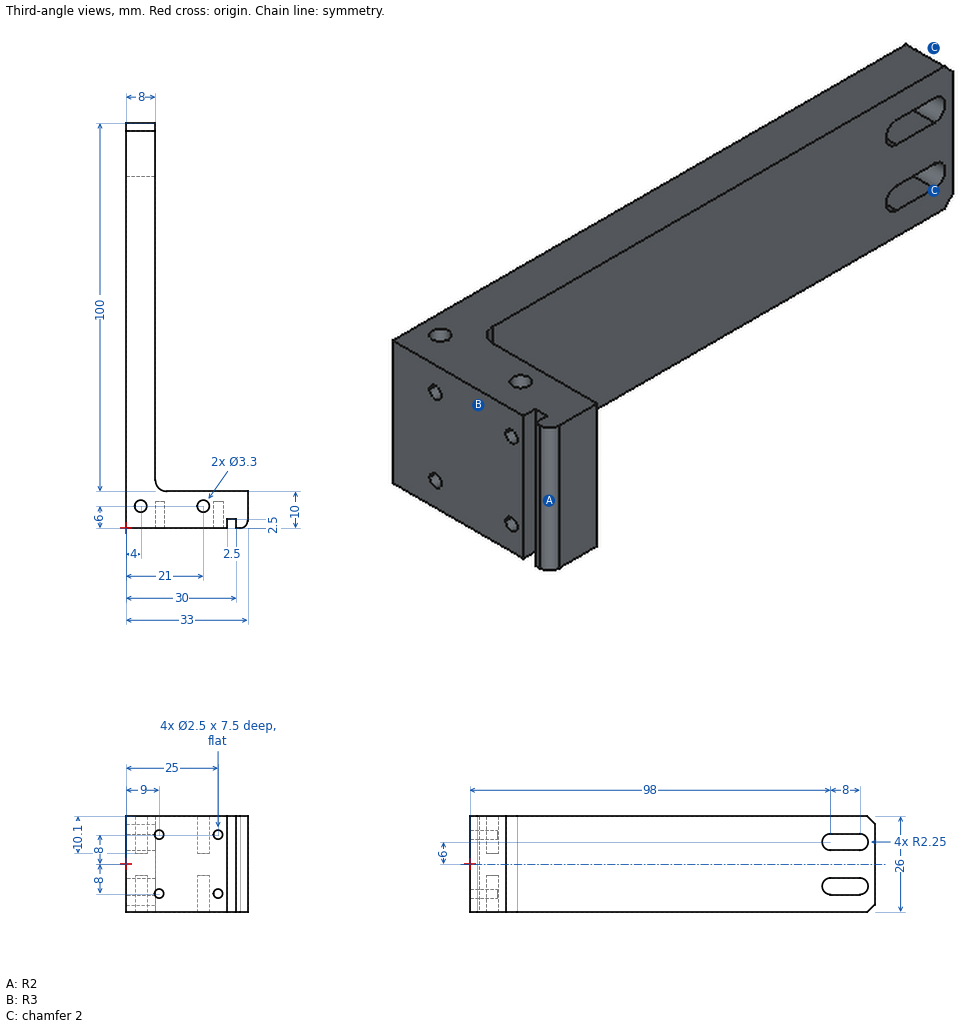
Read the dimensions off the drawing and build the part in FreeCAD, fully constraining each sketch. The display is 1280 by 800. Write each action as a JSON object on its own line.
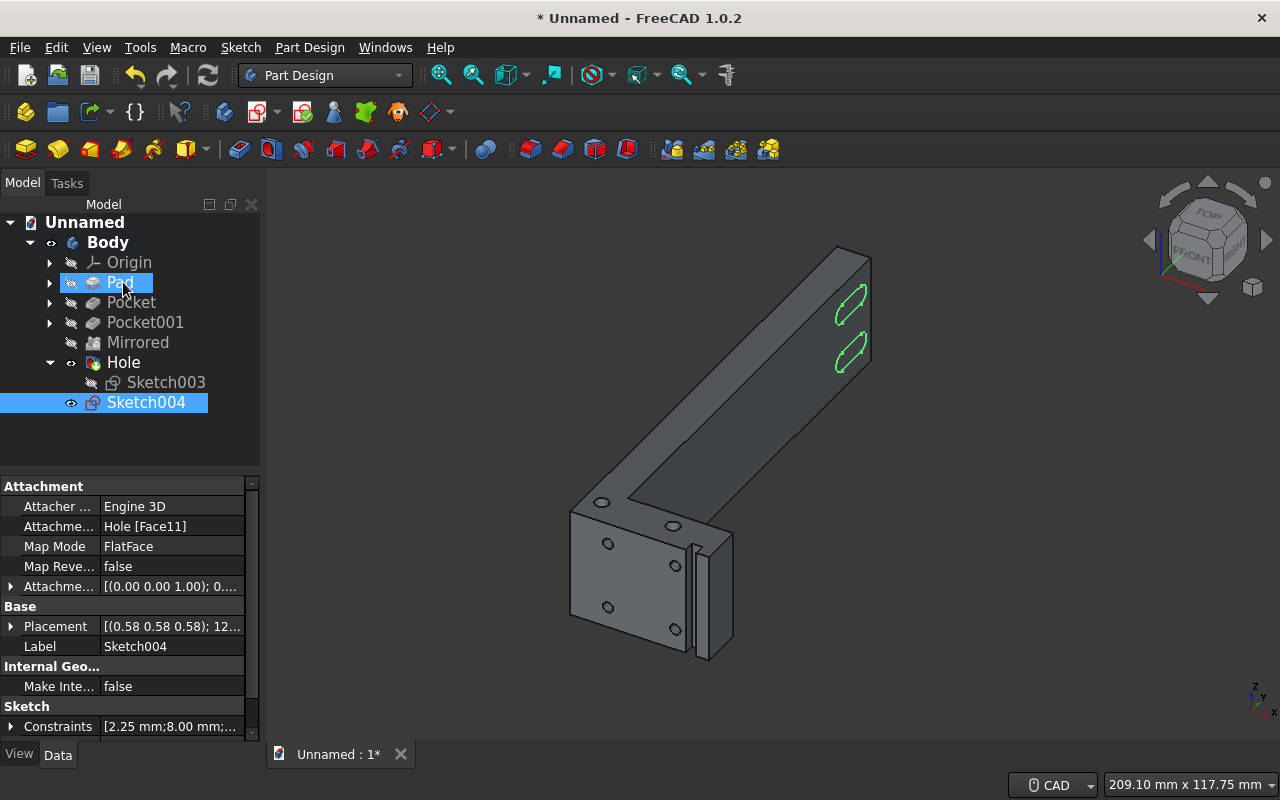
{"action": "left_click", "coordinate": [240, 150]}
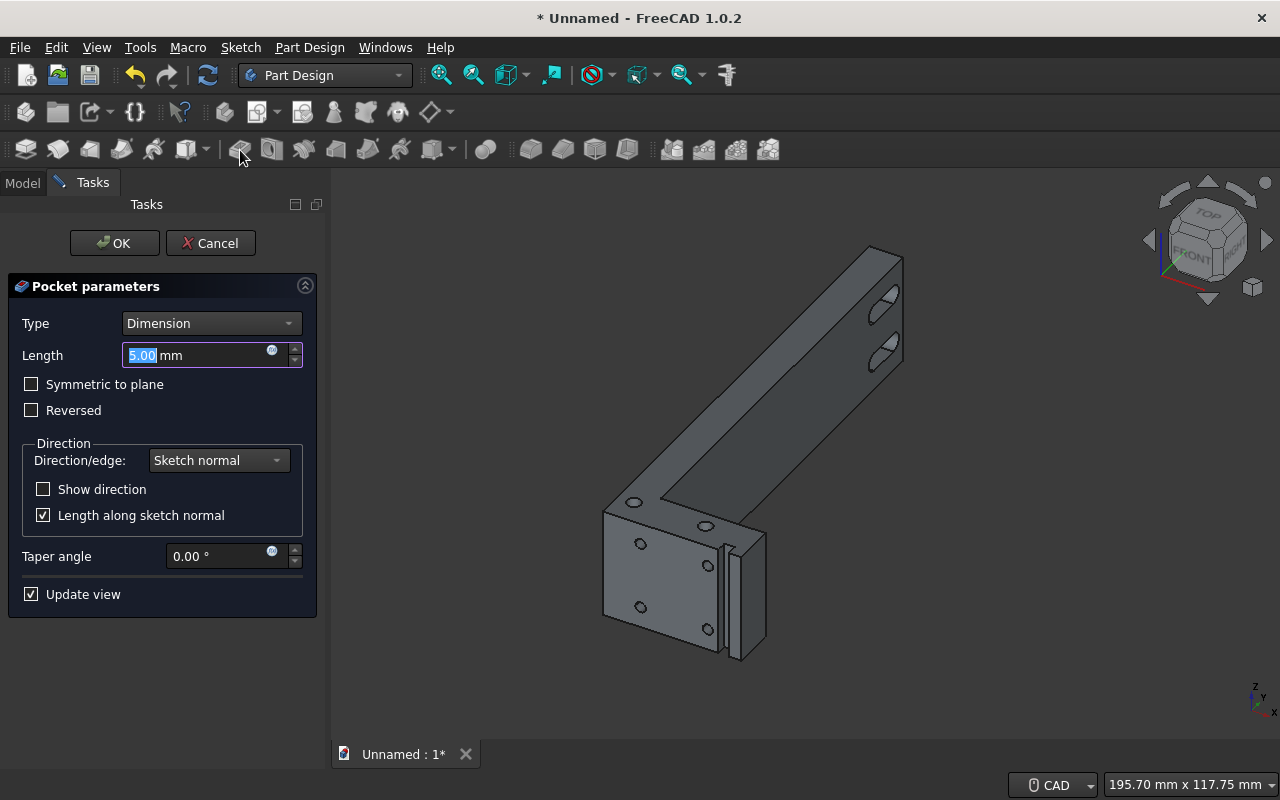
{"action": "left_click", "coordinate": [212, 324]}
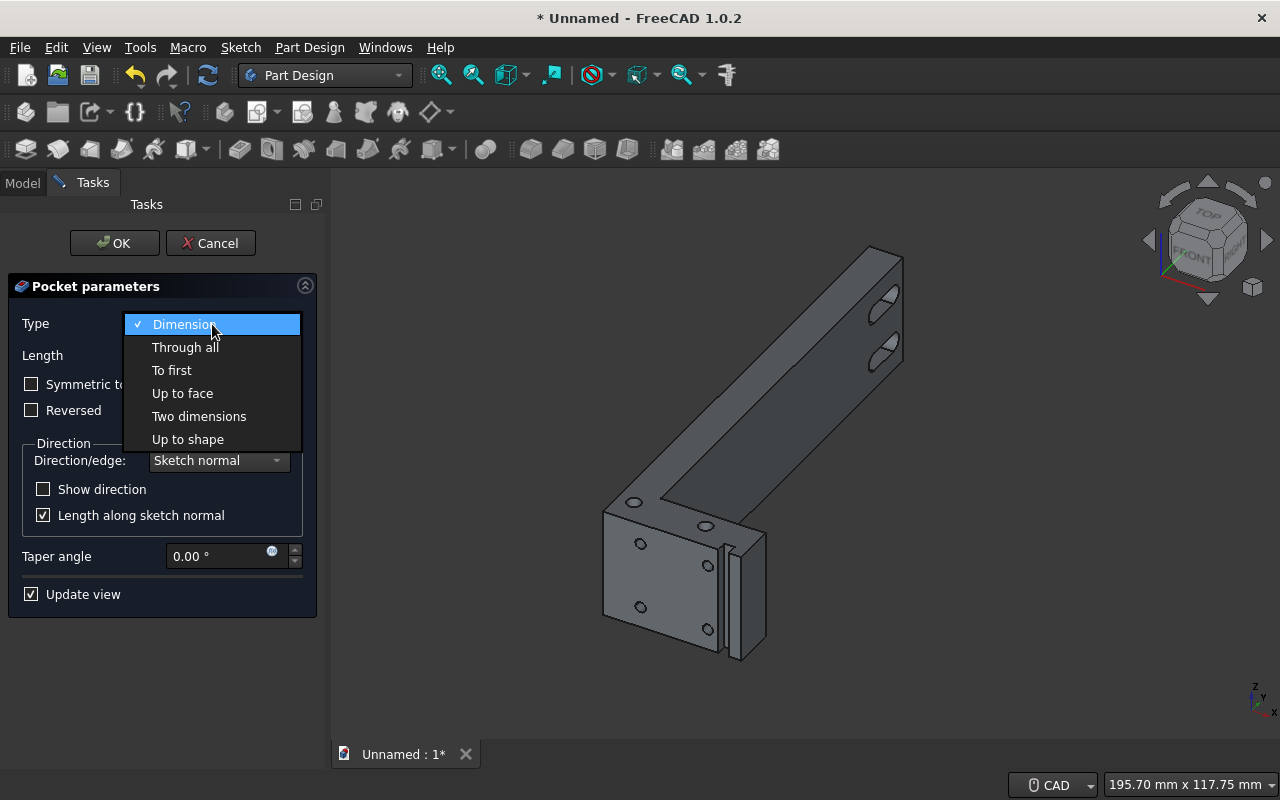
{"action": "left_click", "coordinate": [212, 348]}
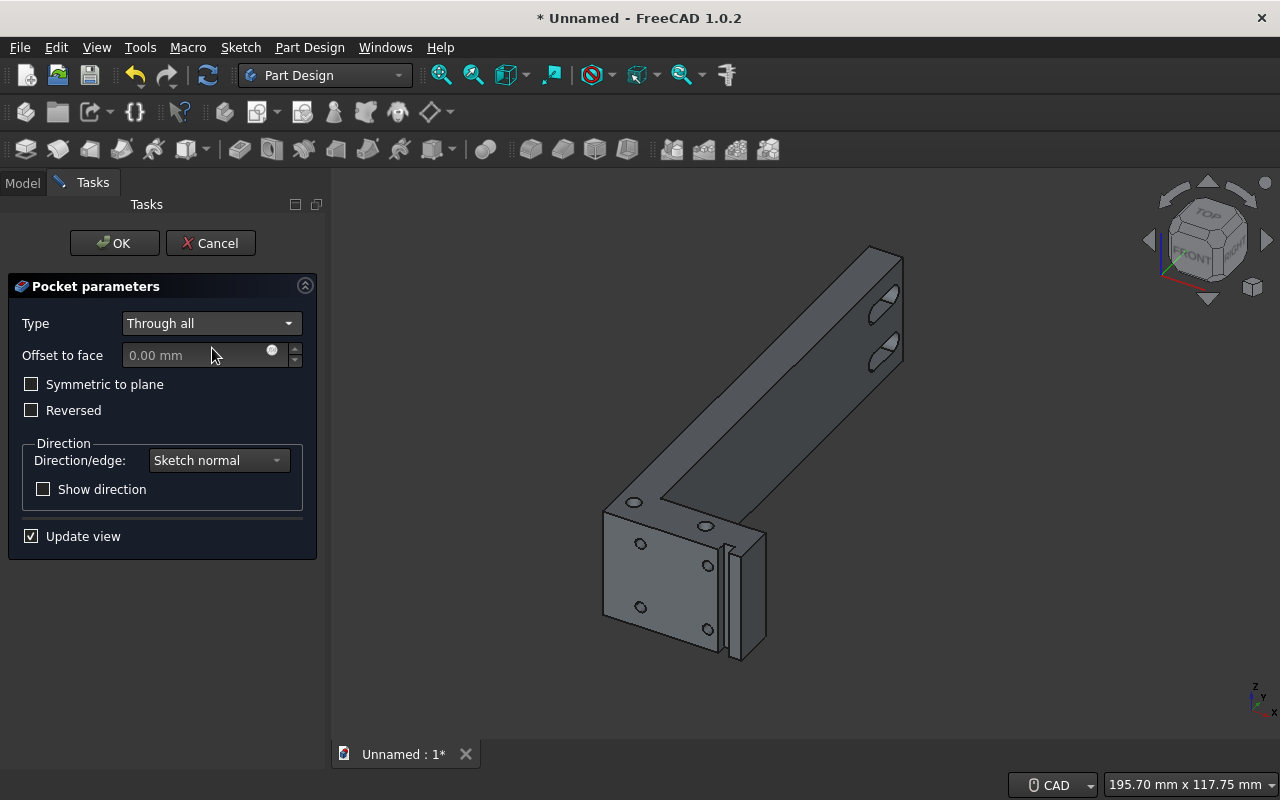
{"action": "left_click", "coordinate": [115, 243]}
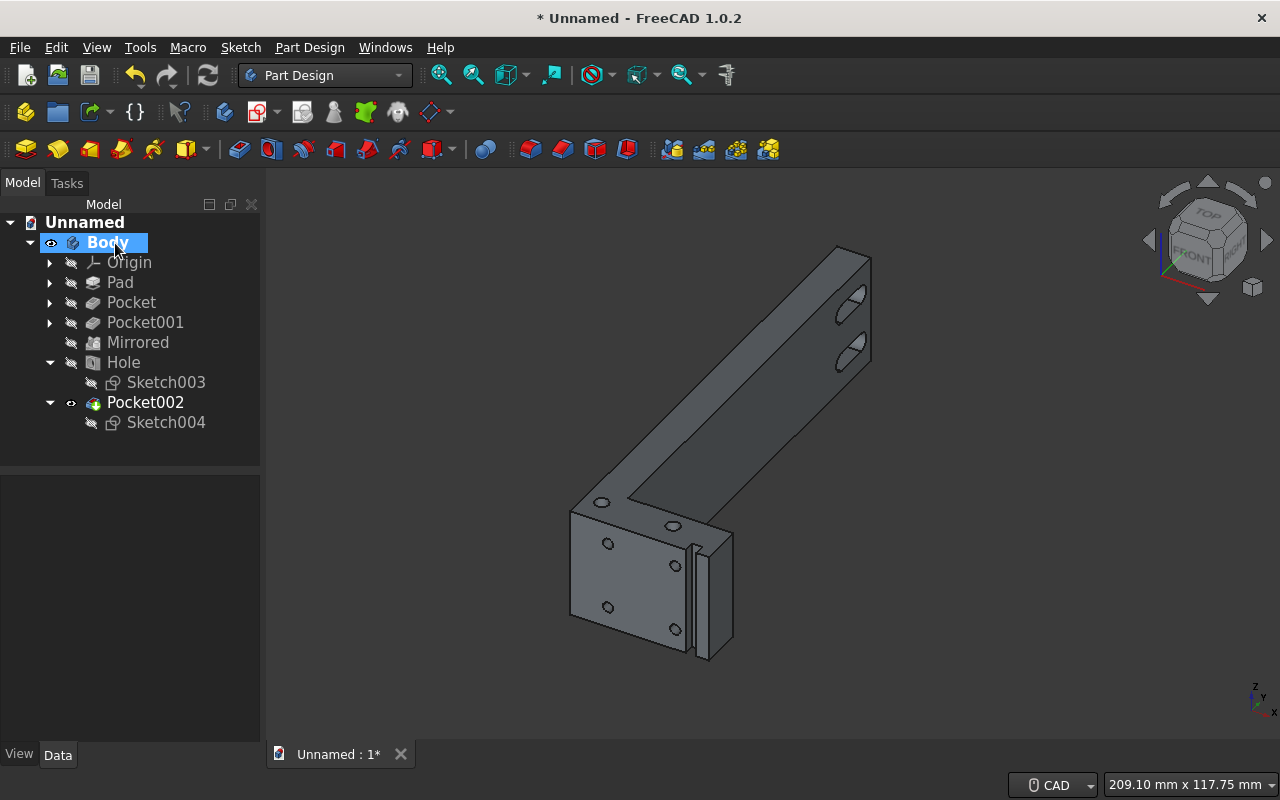
{"action": "left_click", "coordinate": [709, 608]}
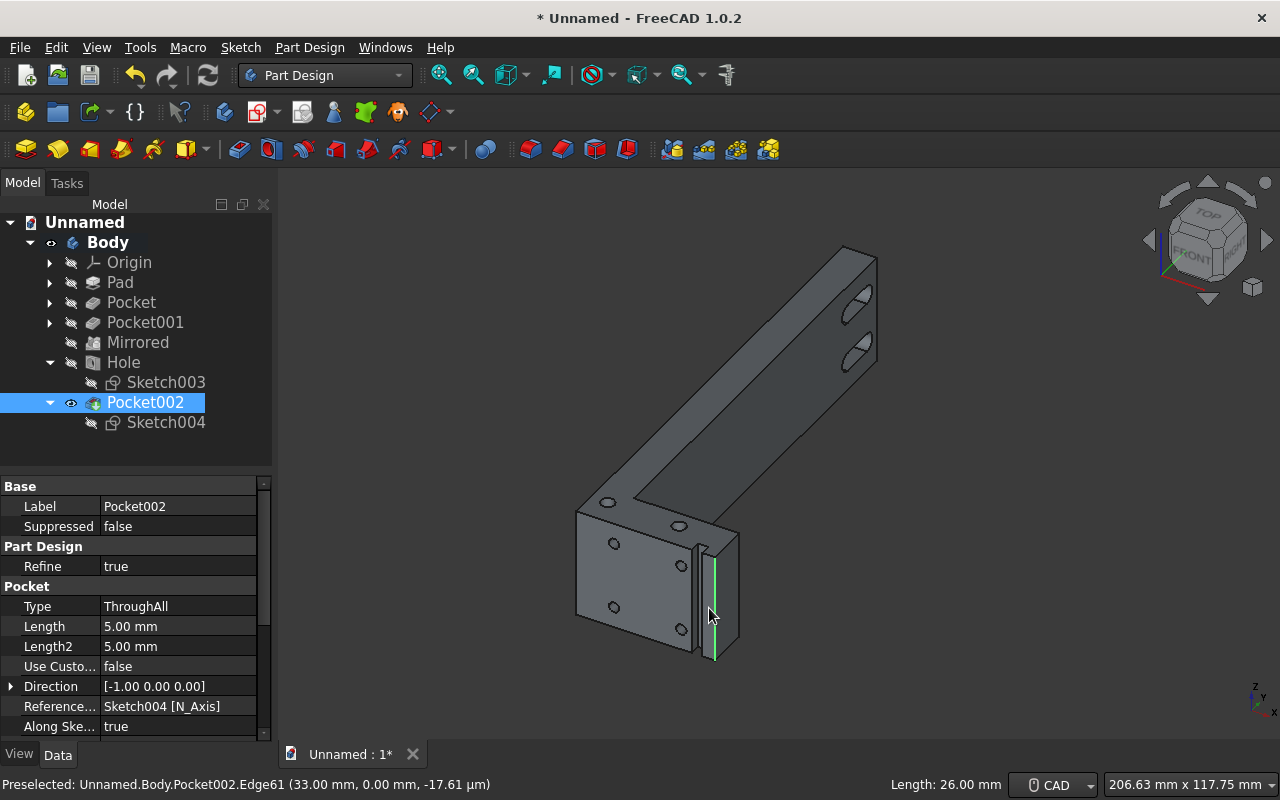
{"action": "left_click", "coordinate": [532, 150]}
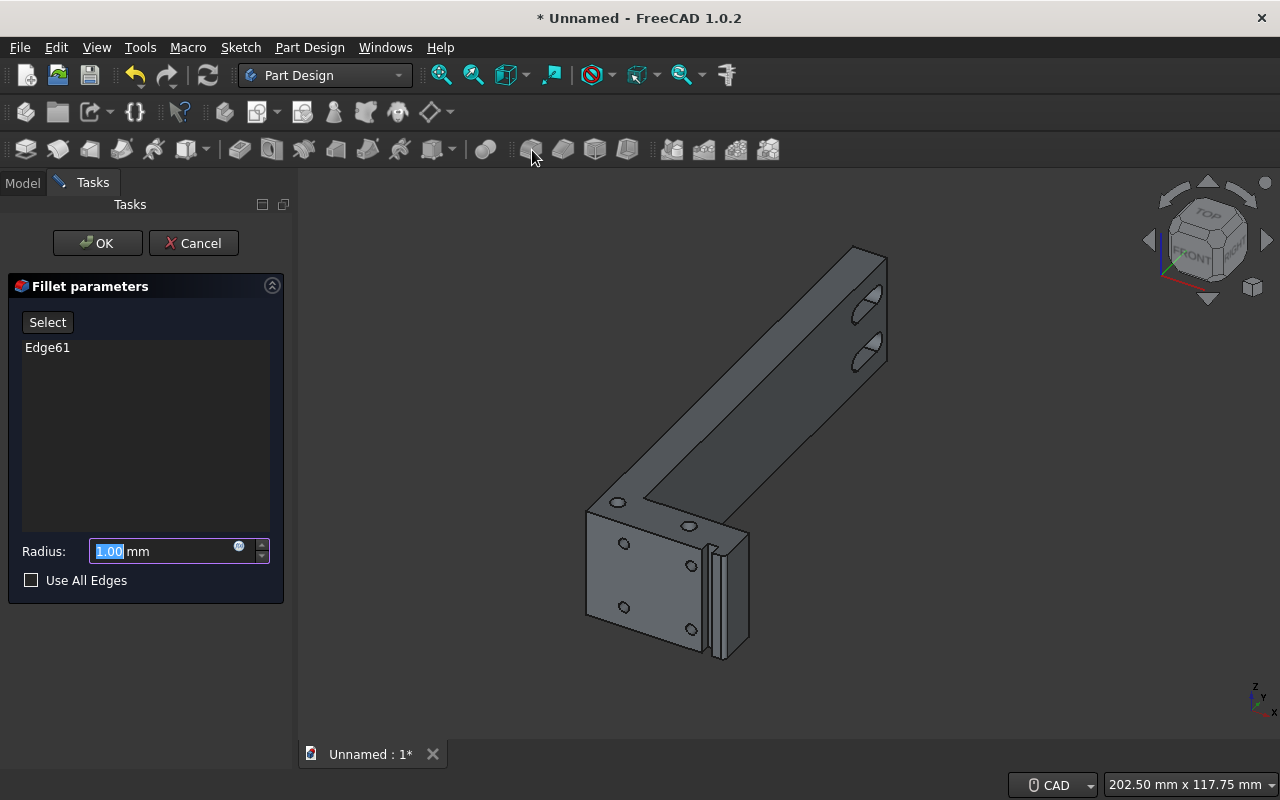
{"action": "type", "text": "2"}
{"action": "key", "text": "Tab"}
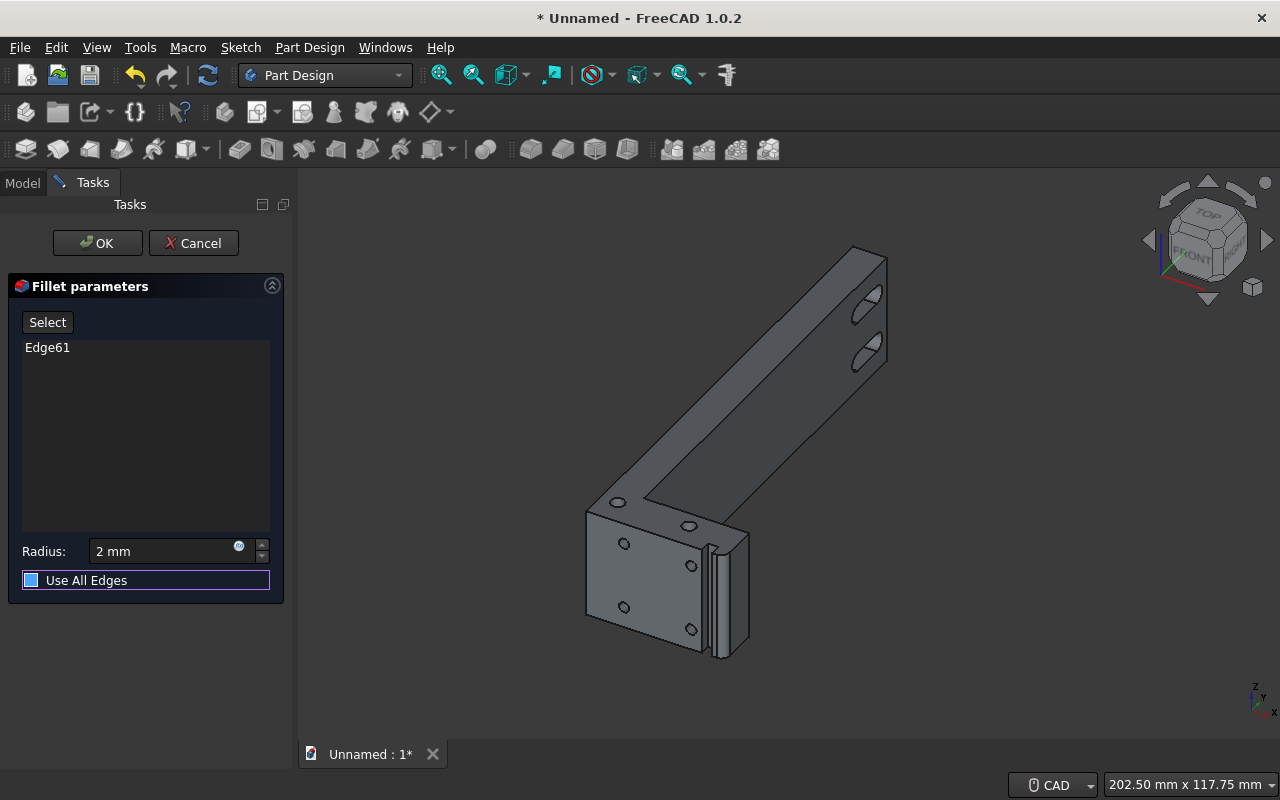
{"action": "left_click", "coordinate": [98, 243]}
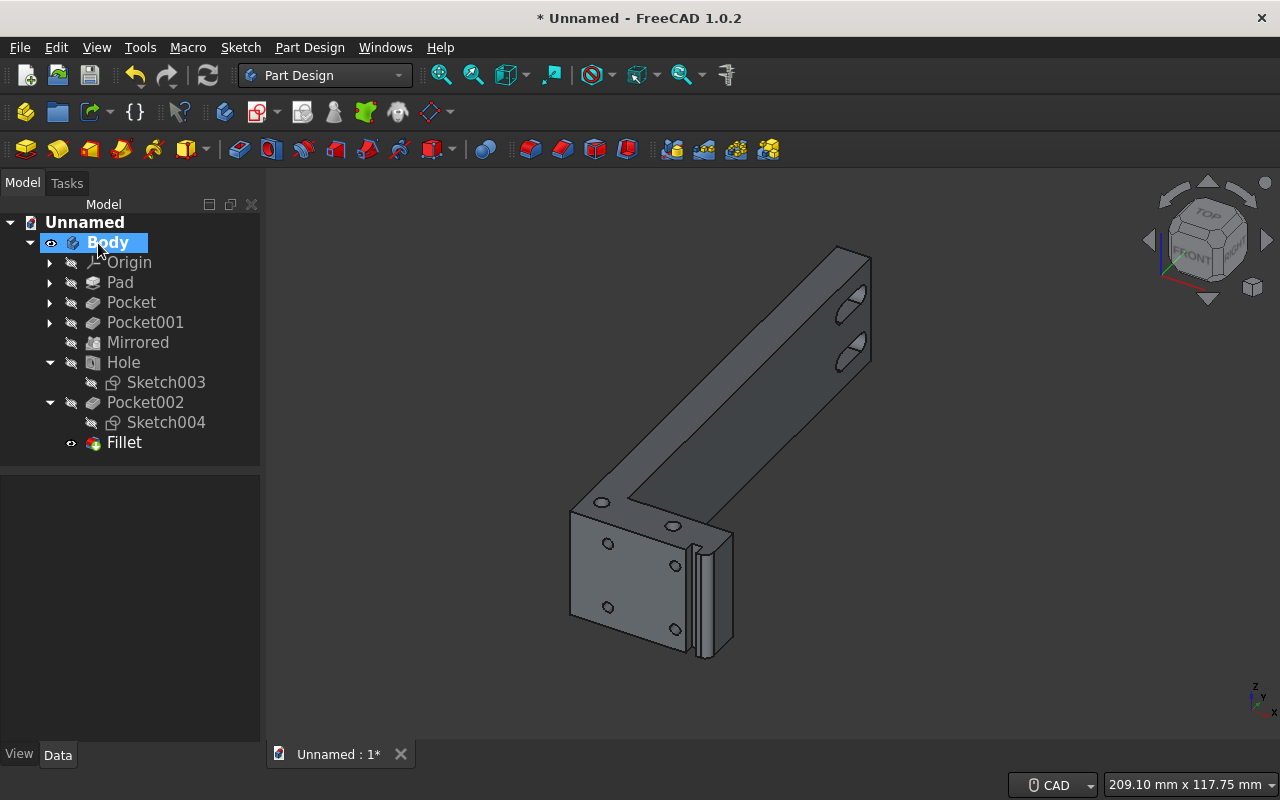
{"action": "key", "text": "0"}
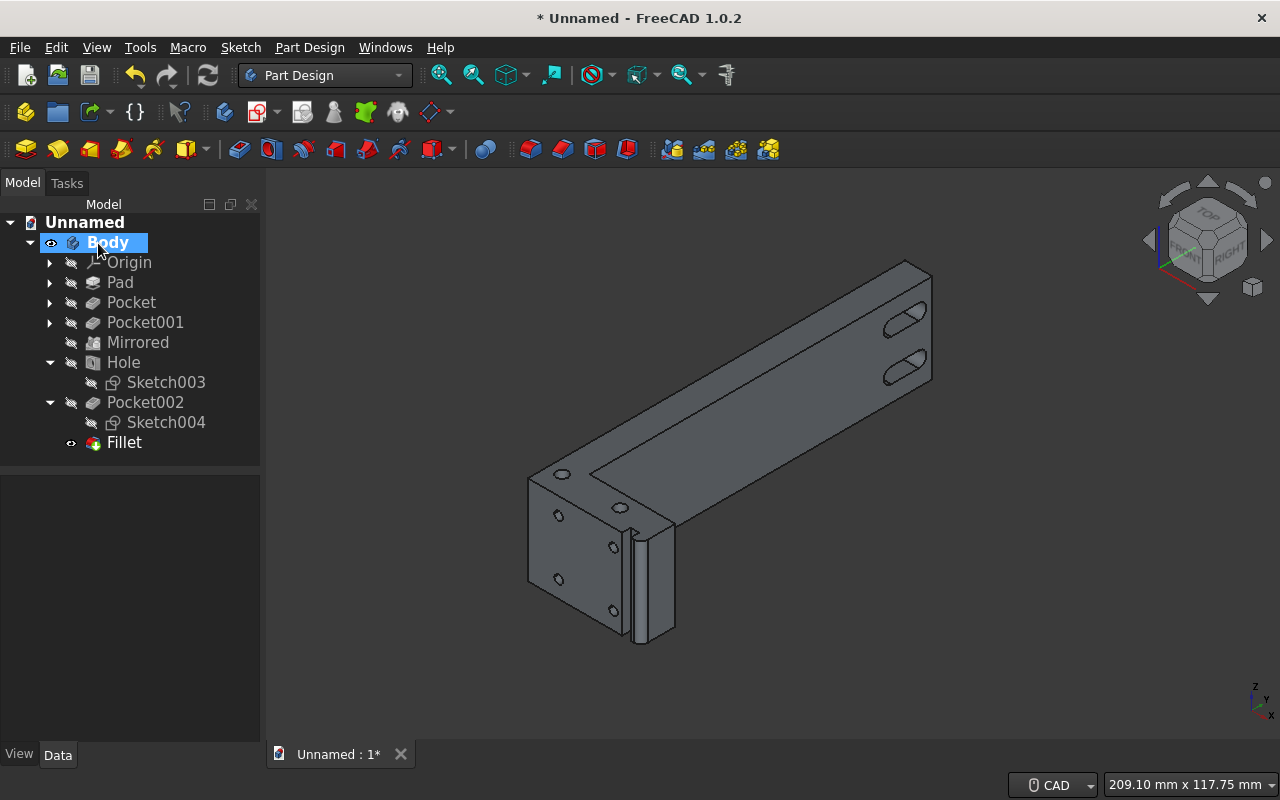
{"action": "key", "text": "2"}